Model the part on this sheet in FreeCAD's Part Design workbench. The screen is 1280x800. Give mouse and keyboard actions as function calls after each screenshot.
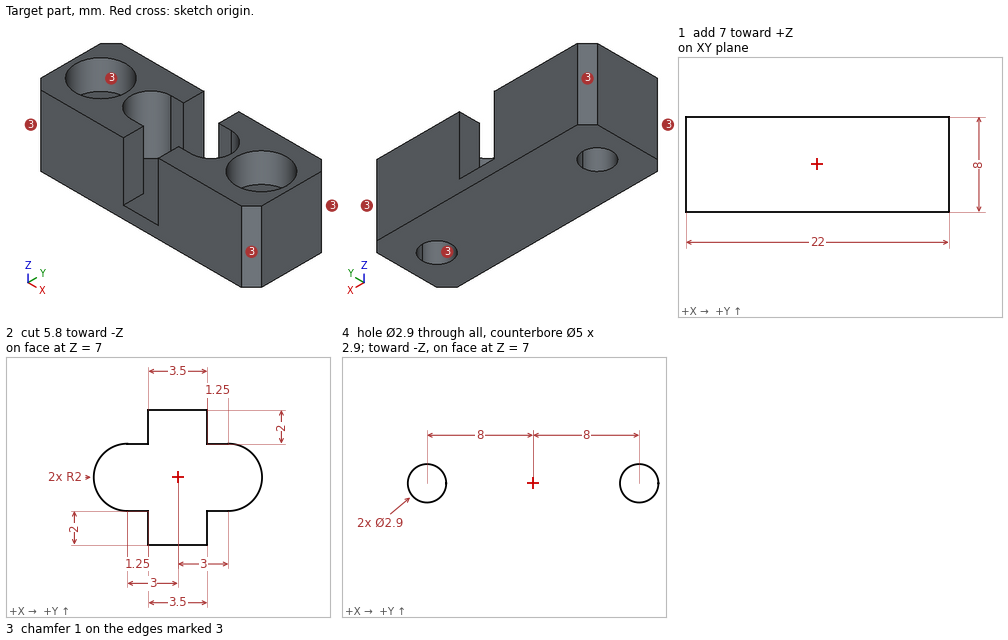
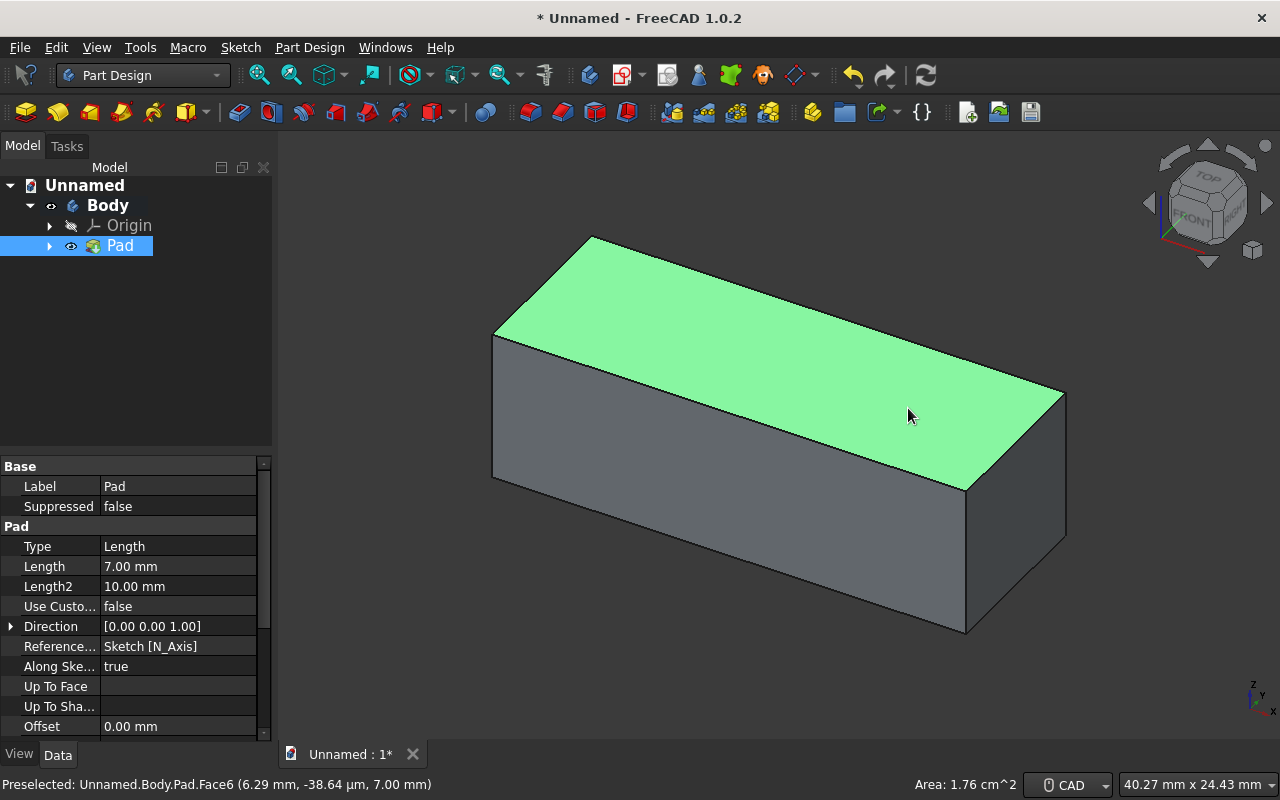
click(622, 76)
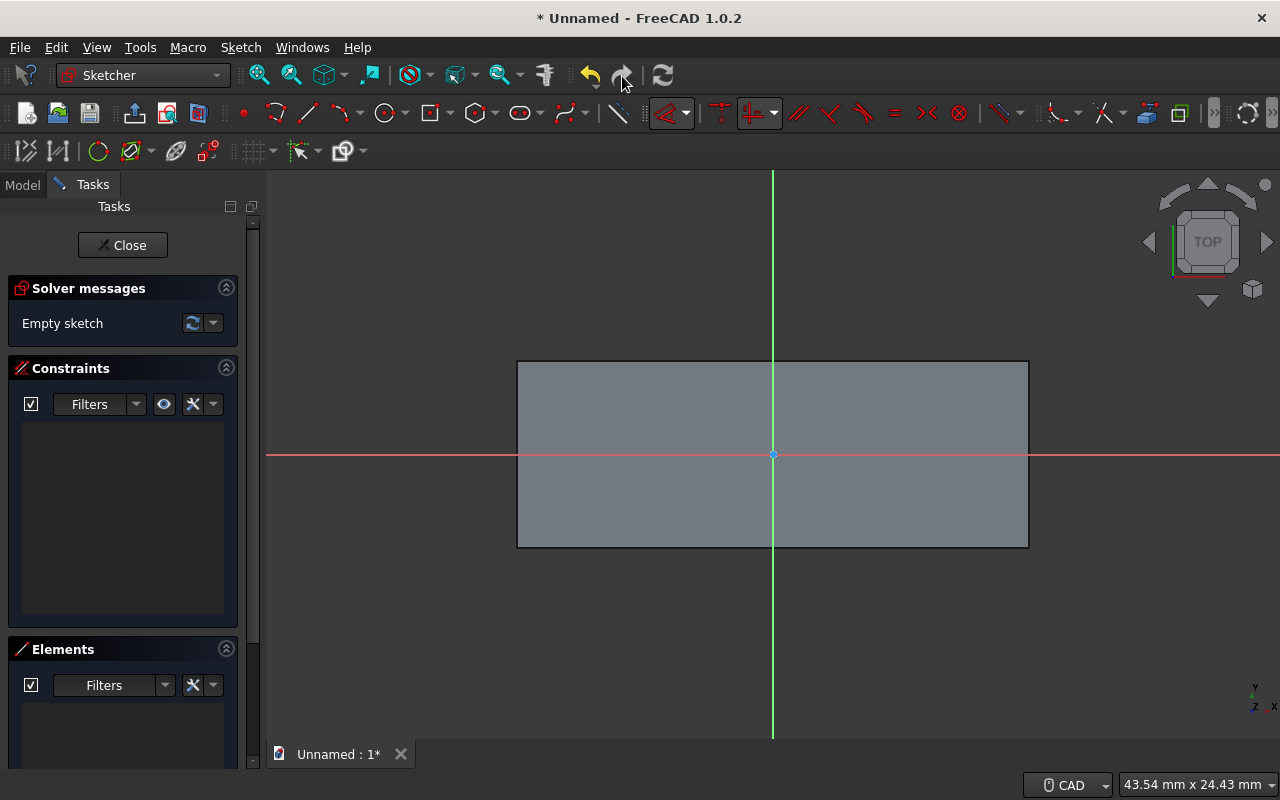
scroll(856, 454, up, 3)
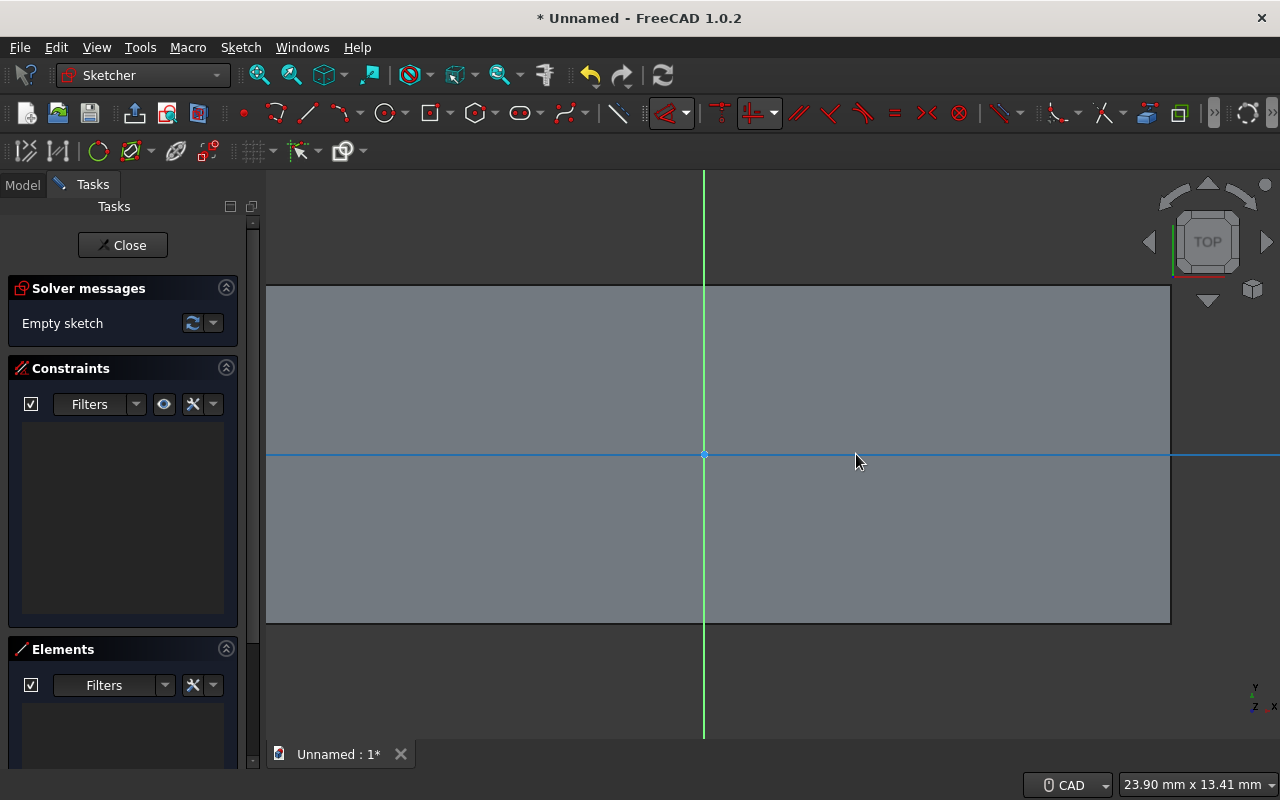
click(276, 114)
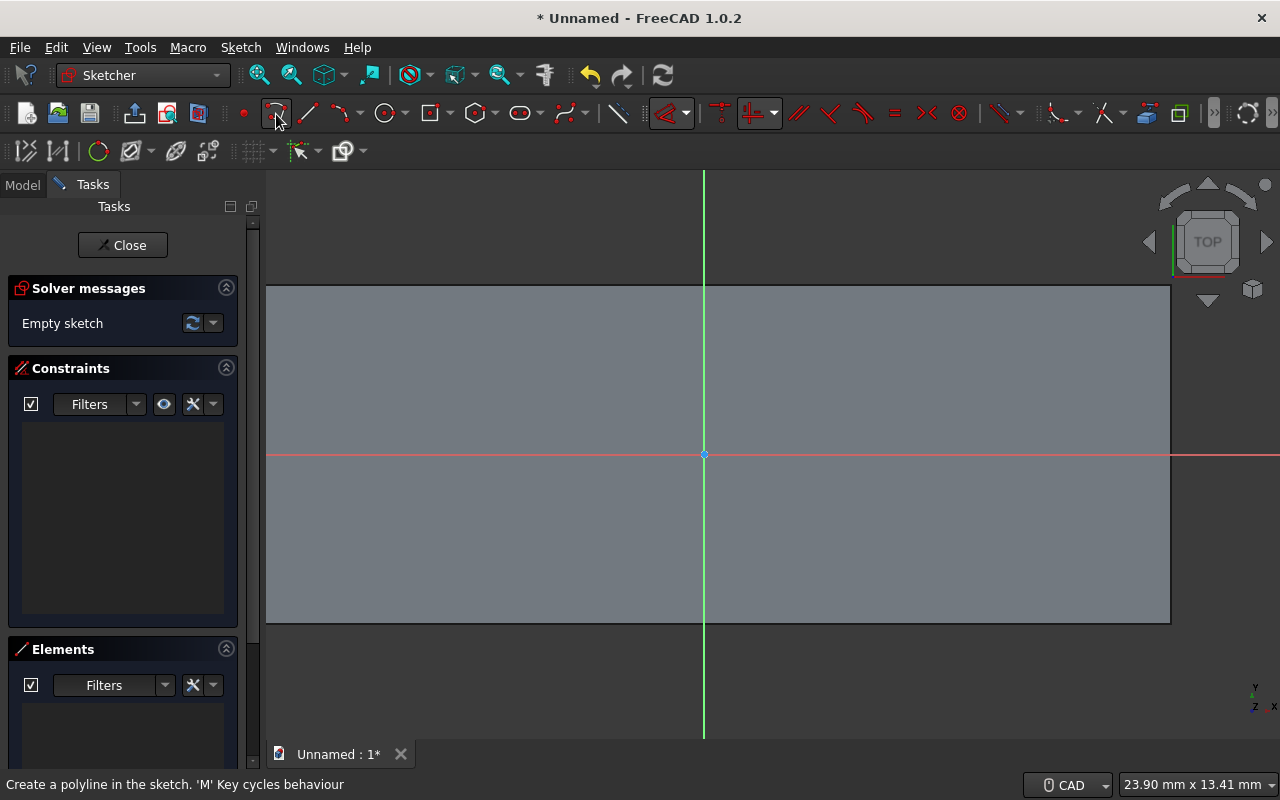
click(577, 539)
click(630, 539)
click(630, 624)
click(779, 624)
click(779, 539)
click(832, 539)
right_click(832, 539)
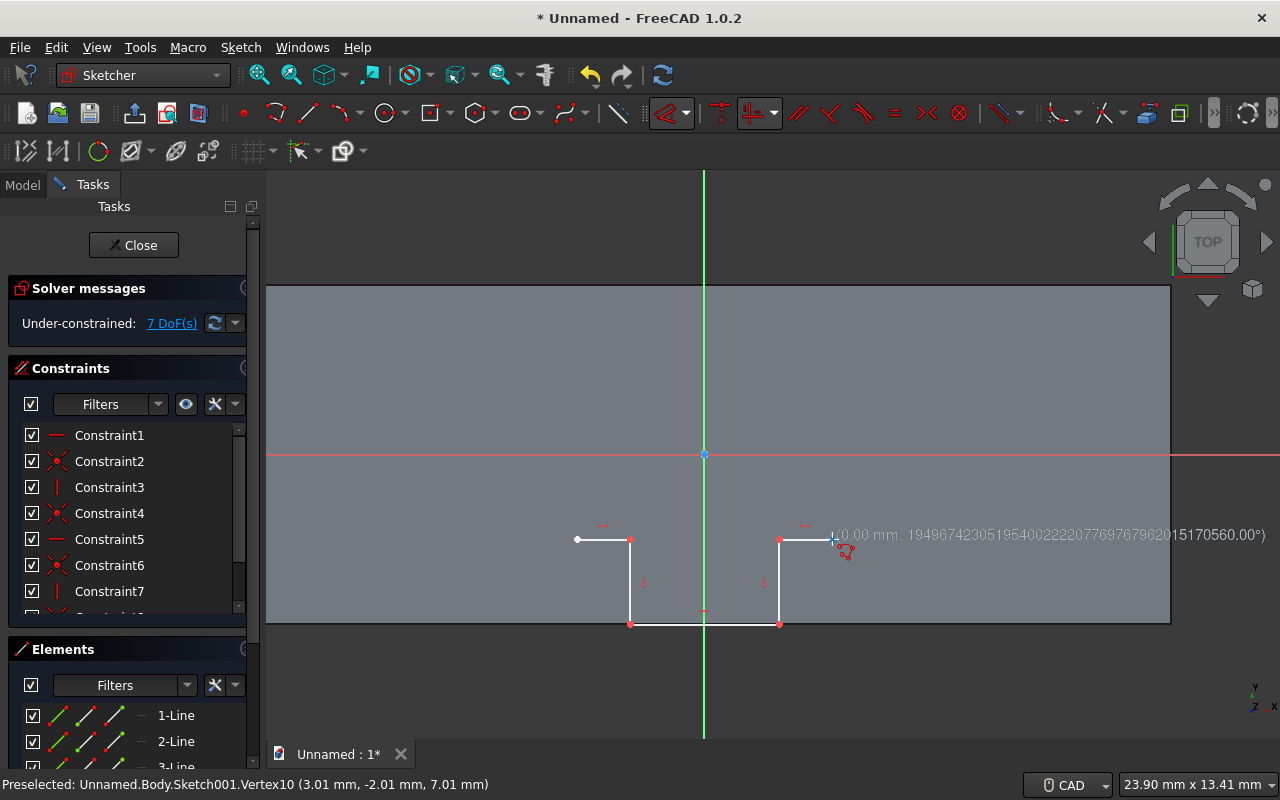
click(832, 370)
click(779, 370)
click(779, 285)
click(630, 285)
click(630, 370)
click(577, 370)
right_click(577, 370)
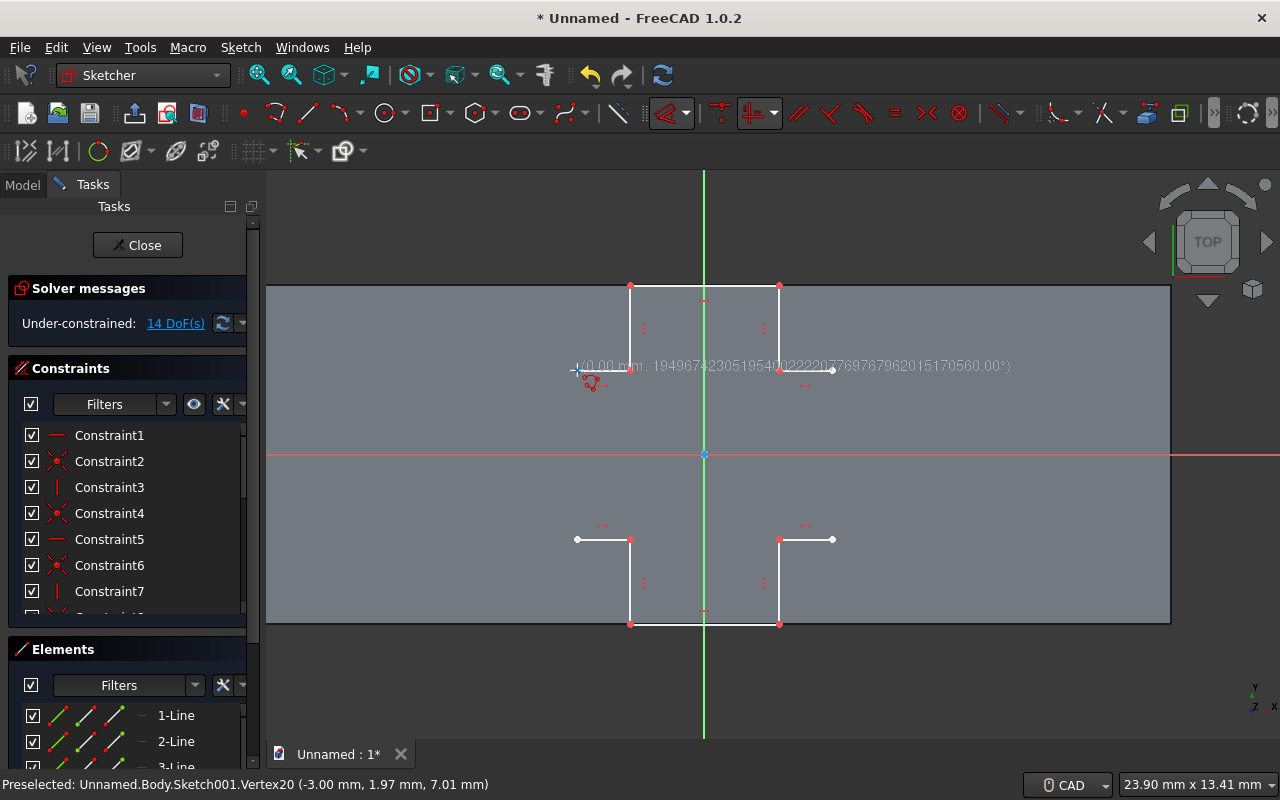
click(340, 114)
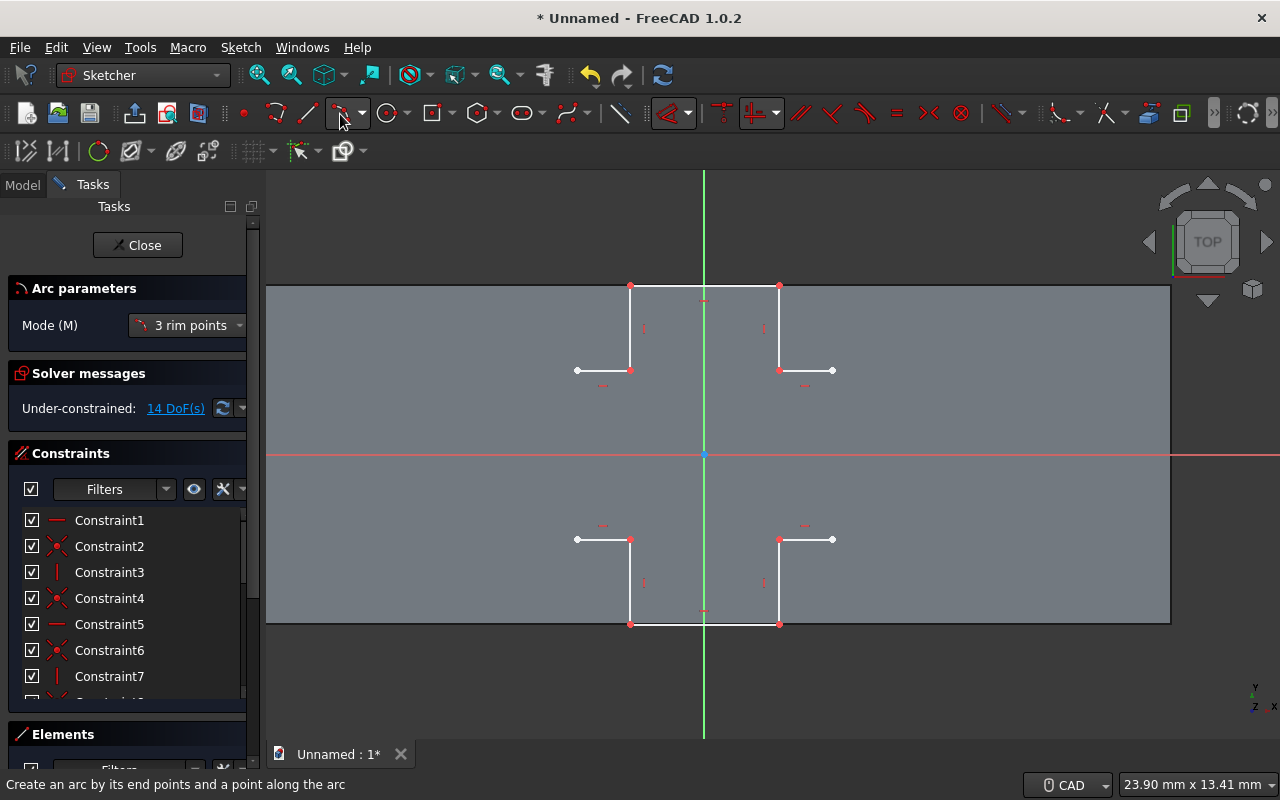
click(832, 540)
click(832, 371)
click(912, 481)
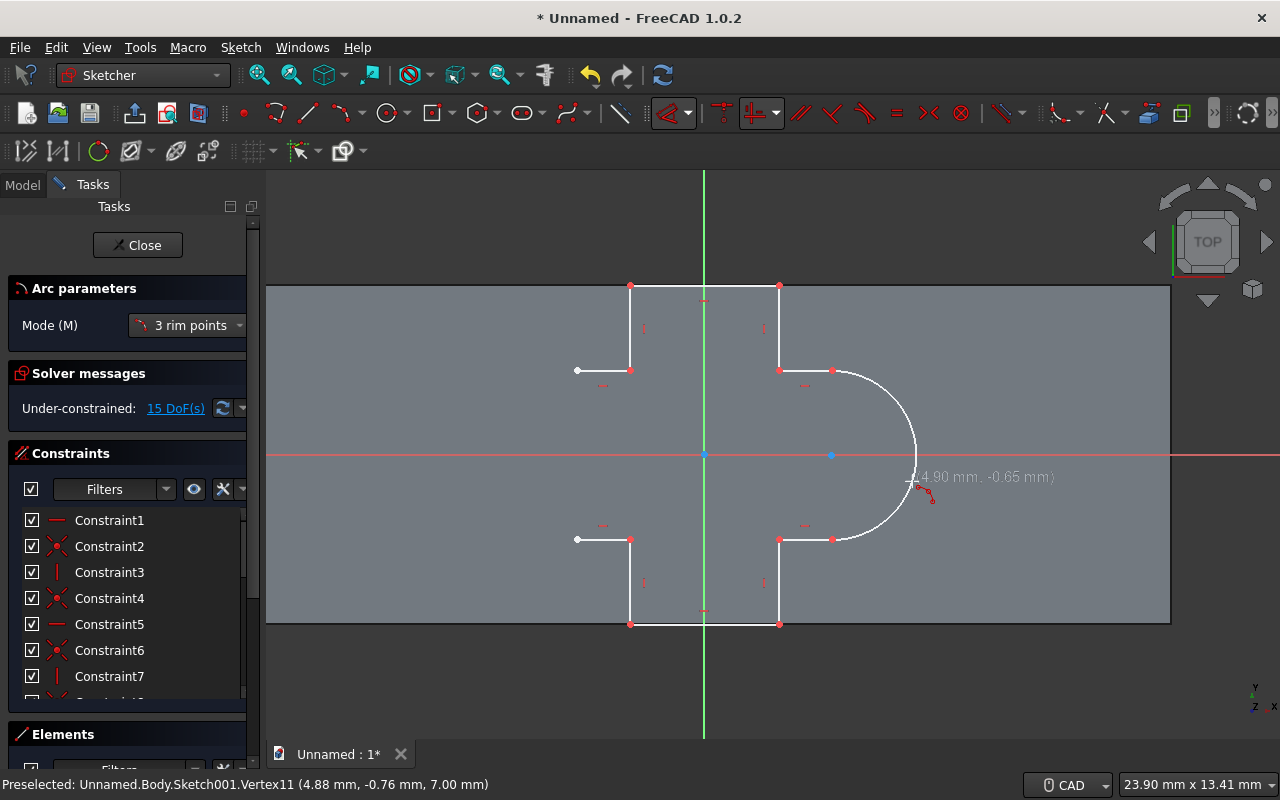
click(577, 371)
click(577, 540)
click(496, 428)
key(Escape)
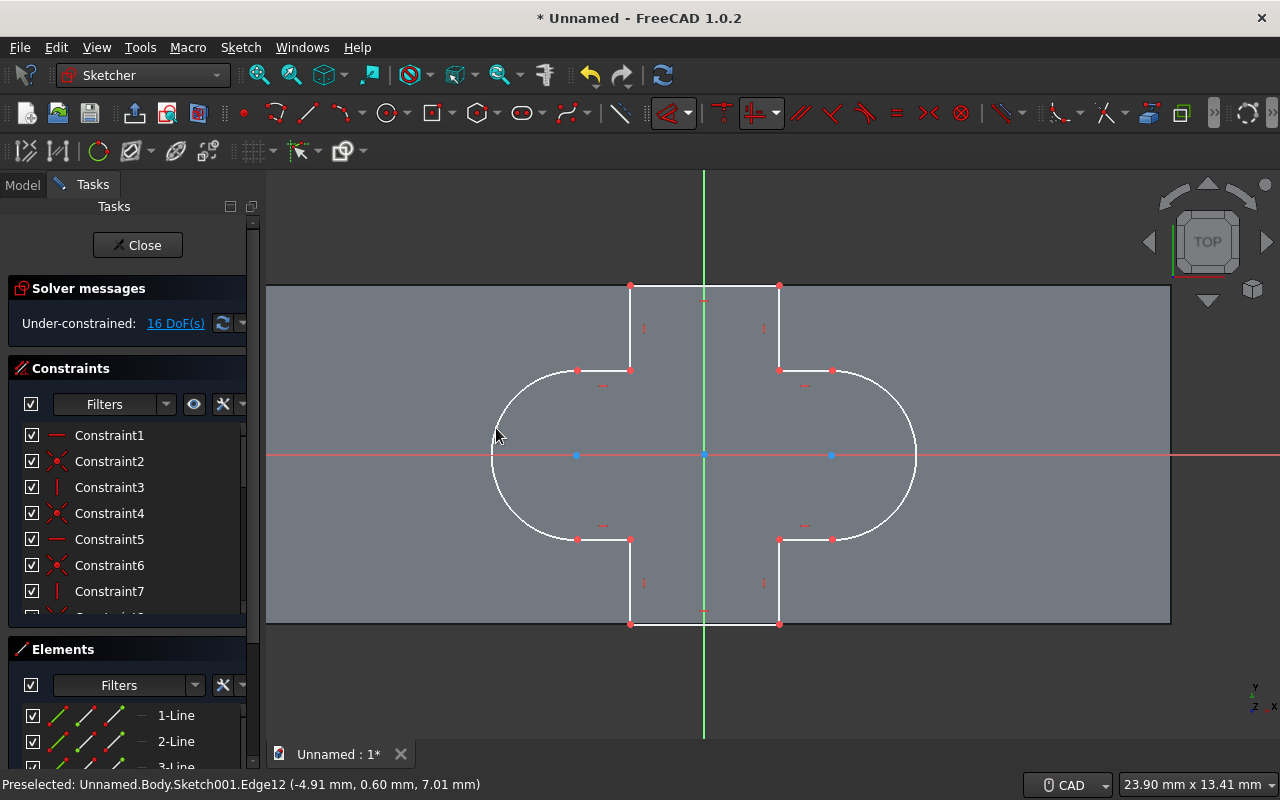
click(593, 540)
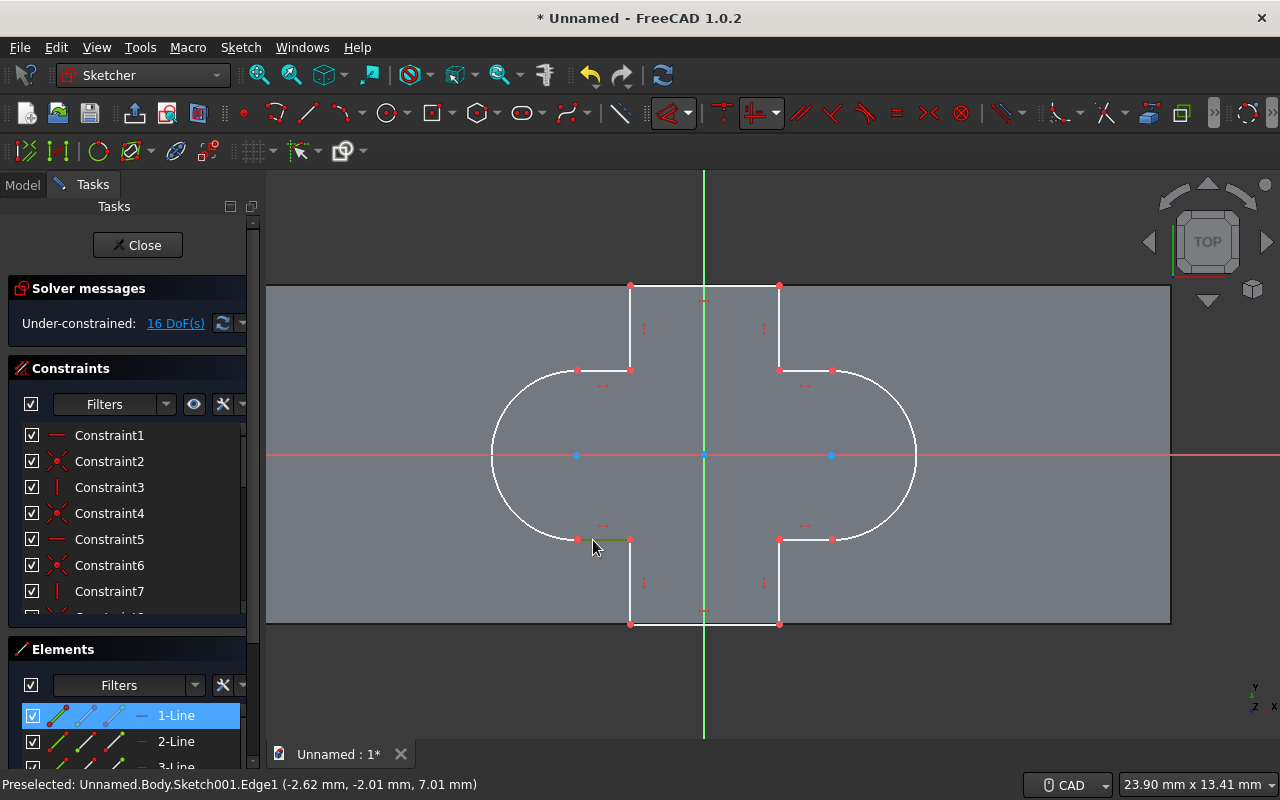
click(508, 406)